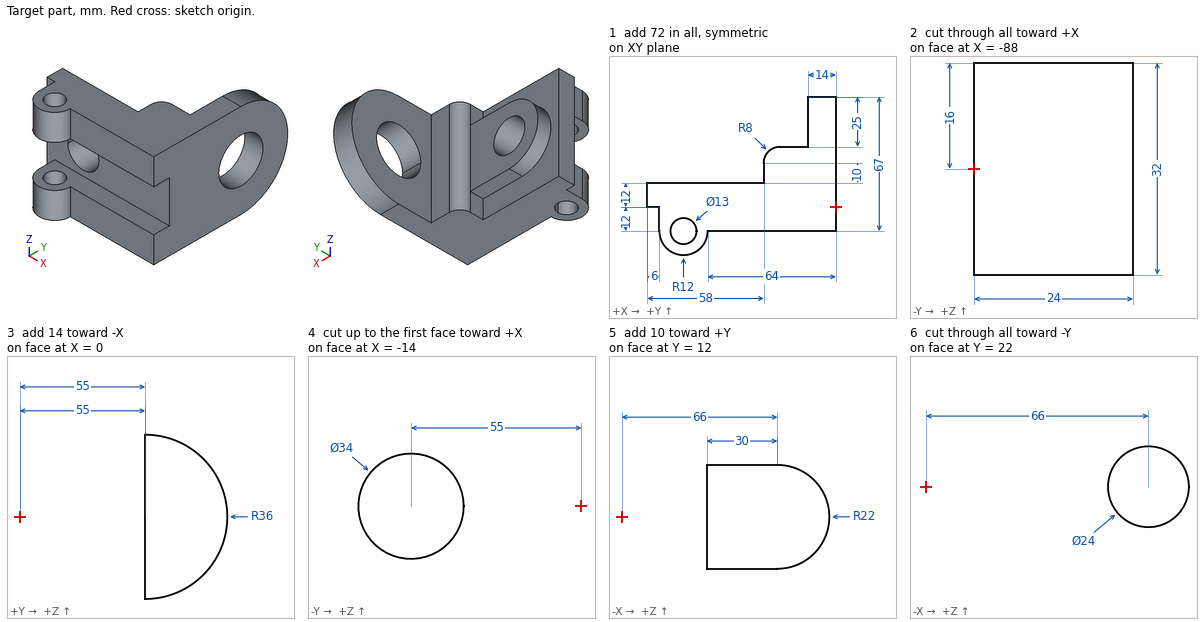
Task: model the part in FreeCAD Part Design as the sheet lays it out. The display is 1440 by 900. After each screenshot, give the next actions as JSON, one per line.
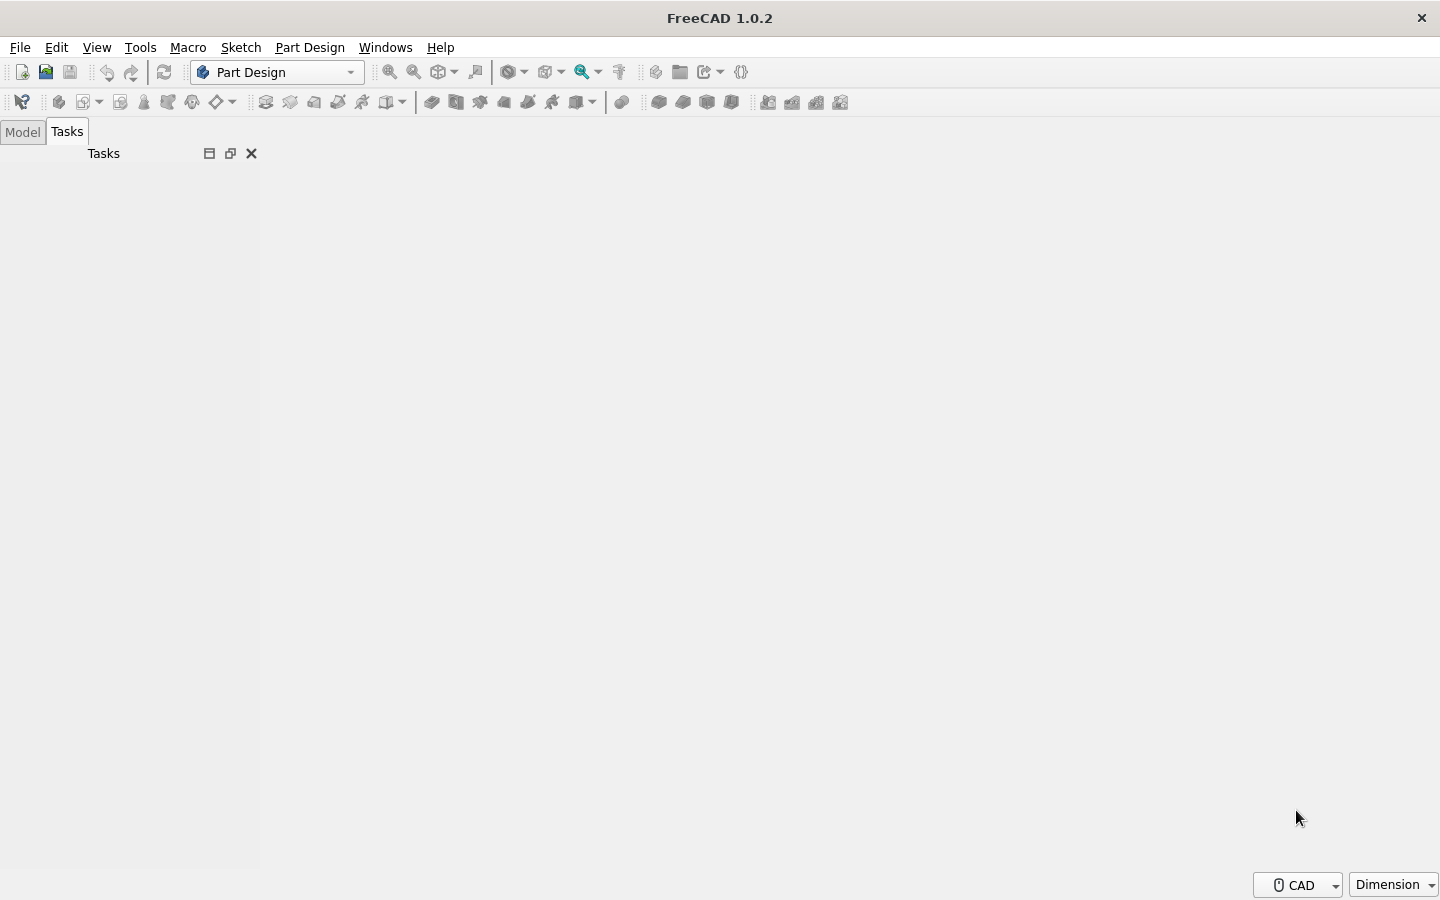
{"action": "left_click", "coordinate": [22, 72]}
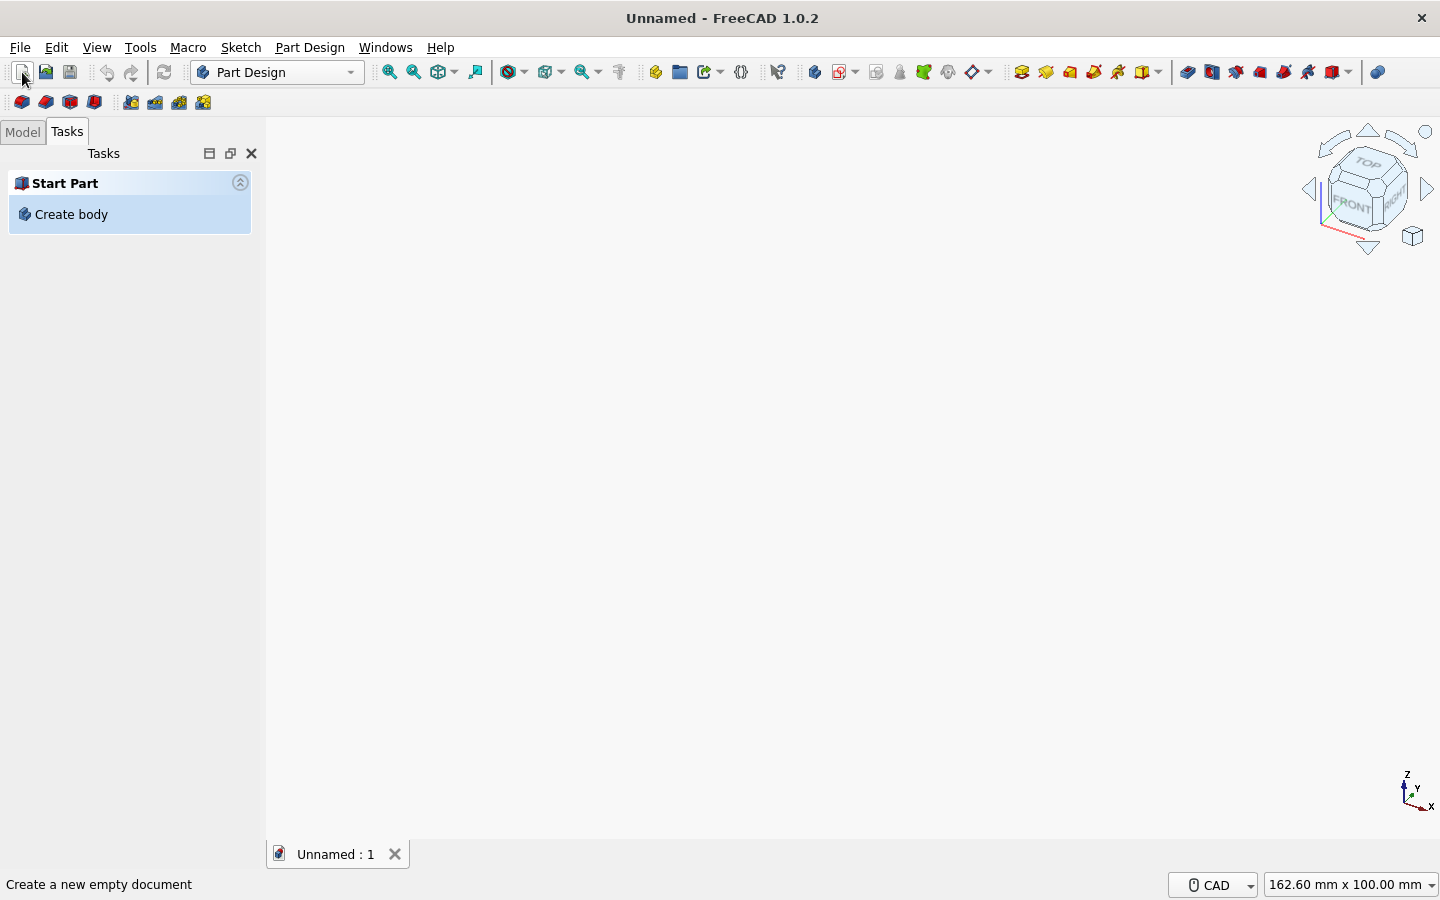
{"action": "left_click", "coordinate": [840, 72]}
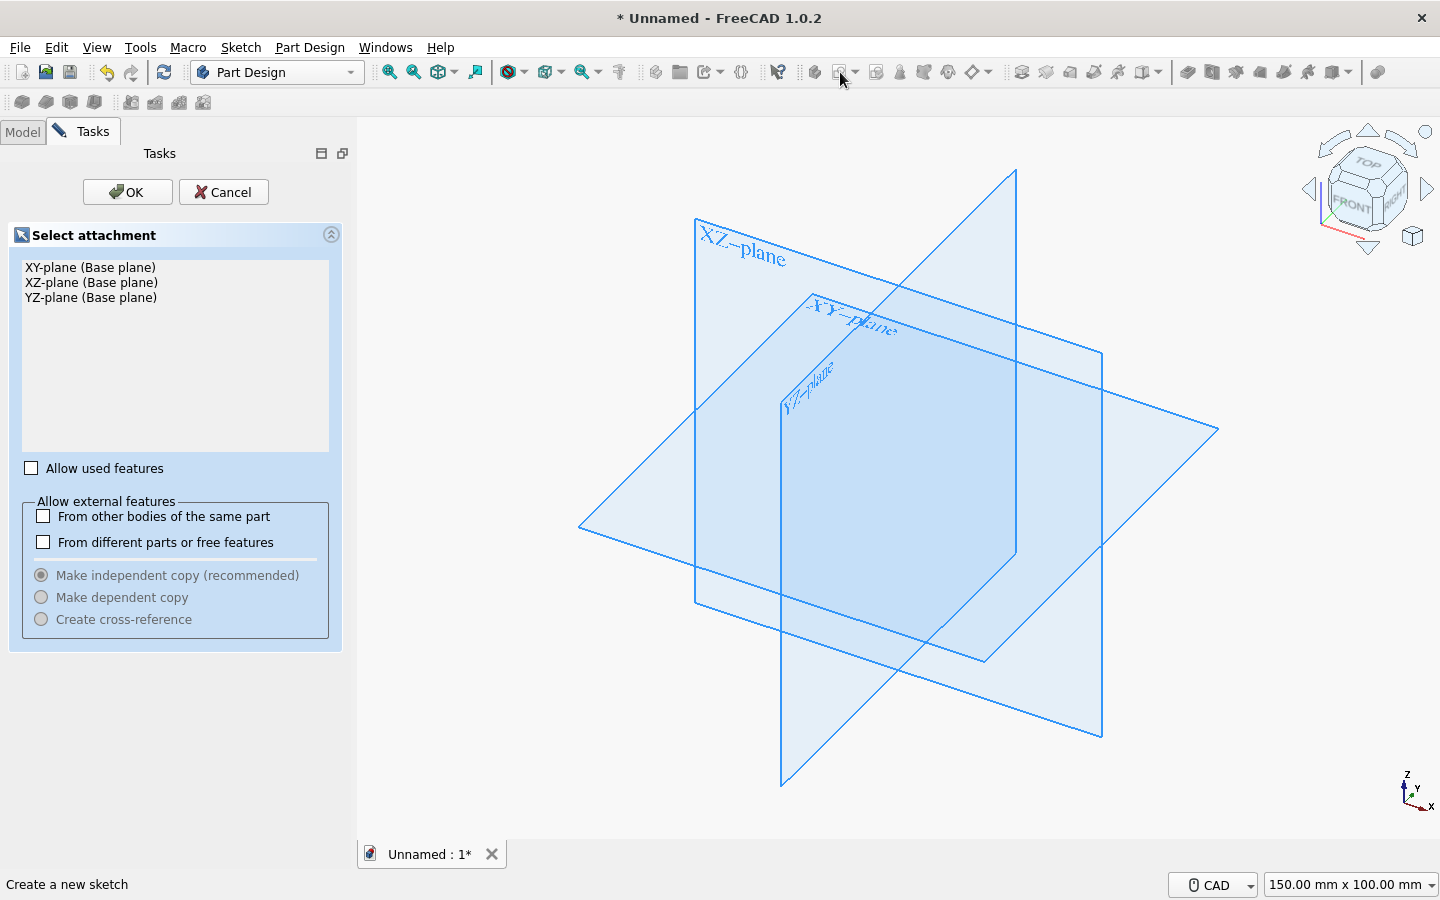
{"action": "left_click", "coordinate": [82, 268]}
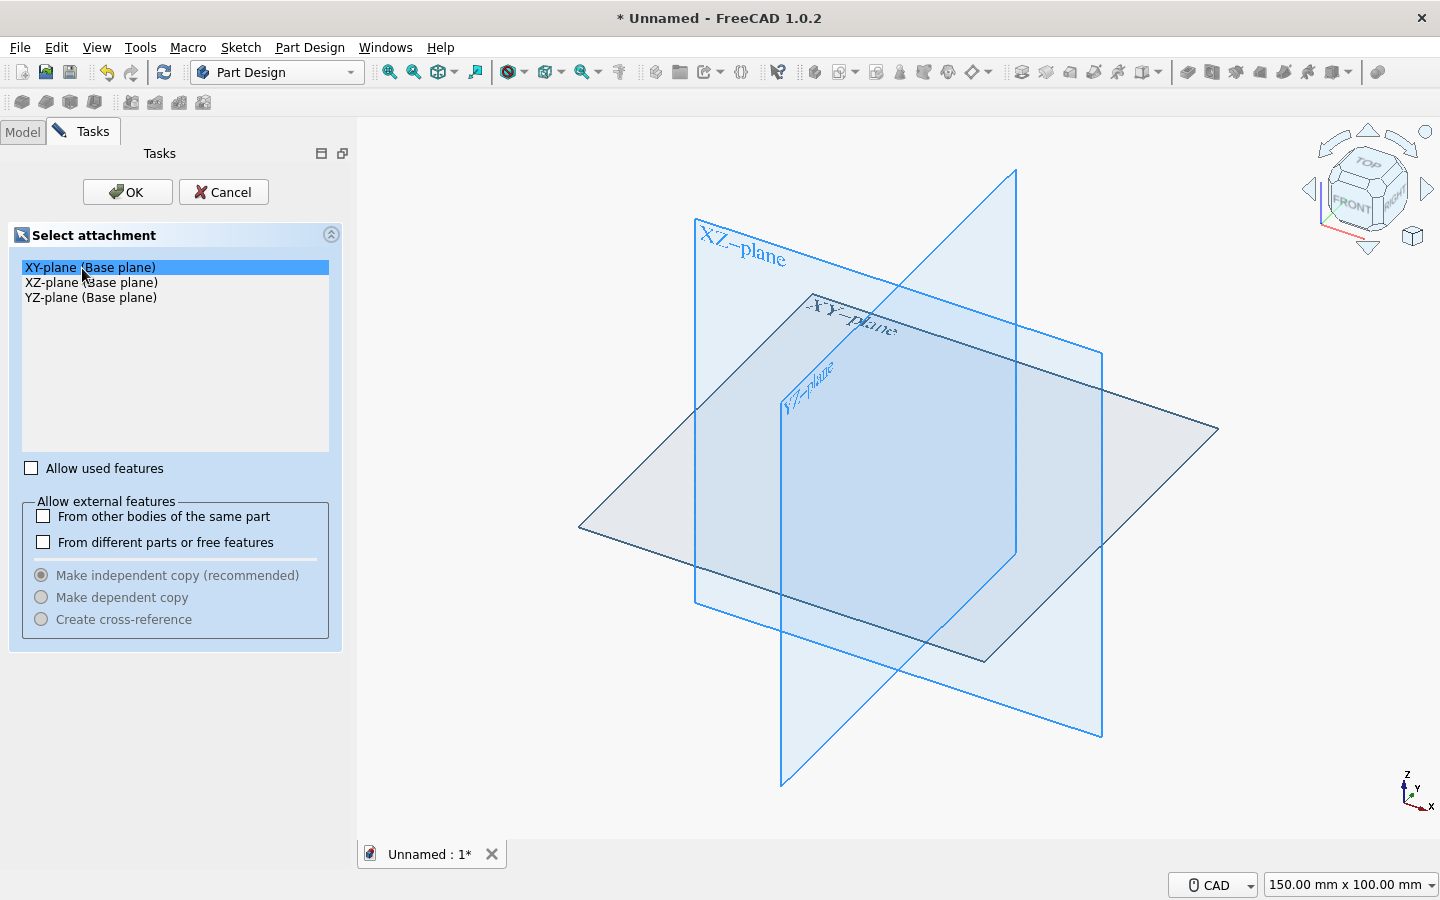
{"action": "left_click", "coordinate": [128, 192]}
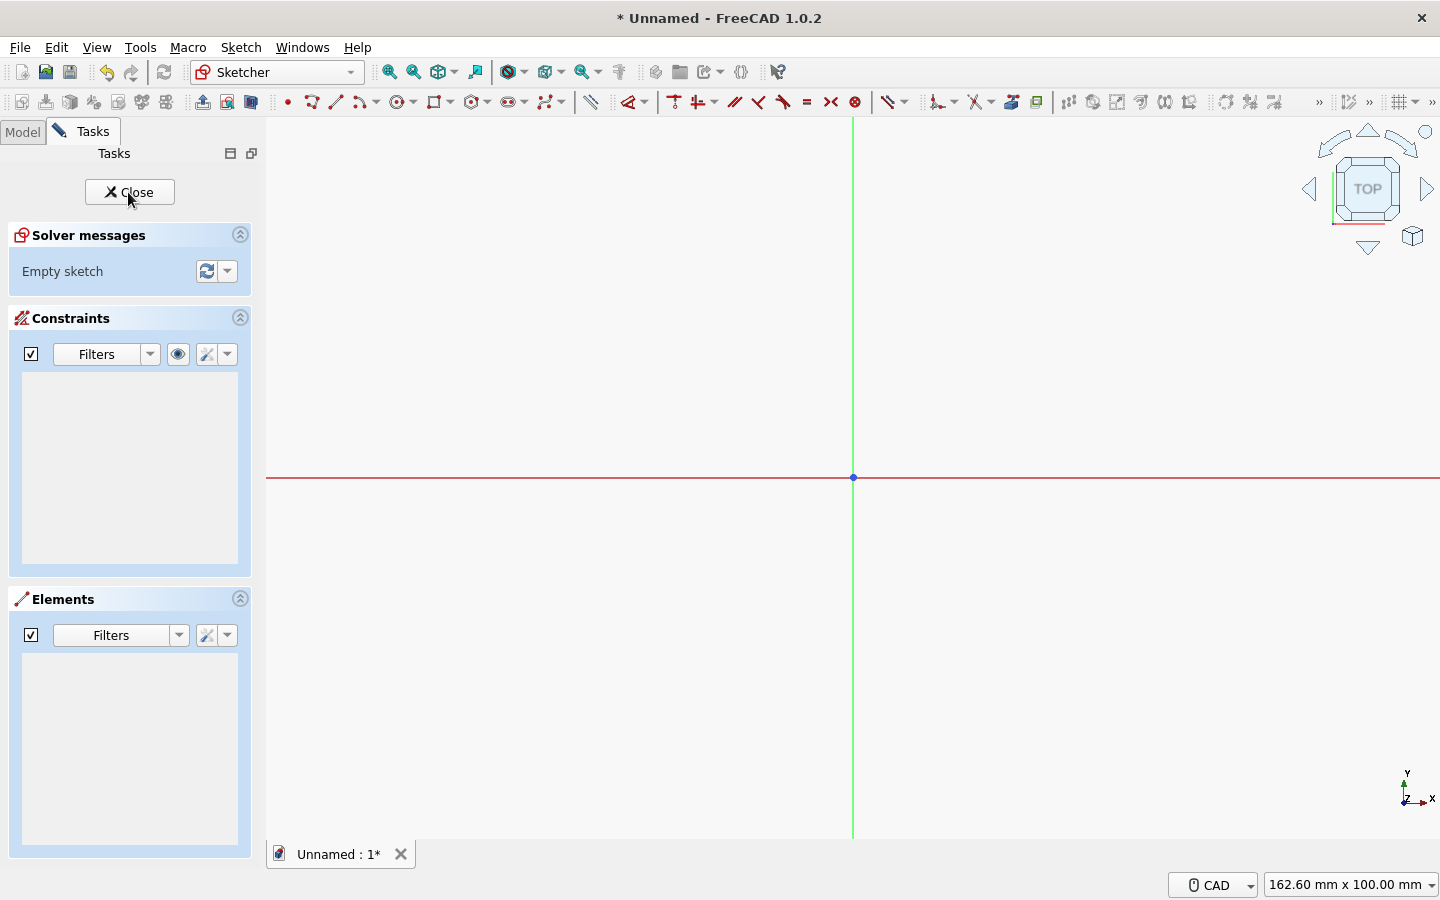
{"action": "scroll", "coordinate": [1275, 811], "scroll_direction": "down", "scroll_amount": 1}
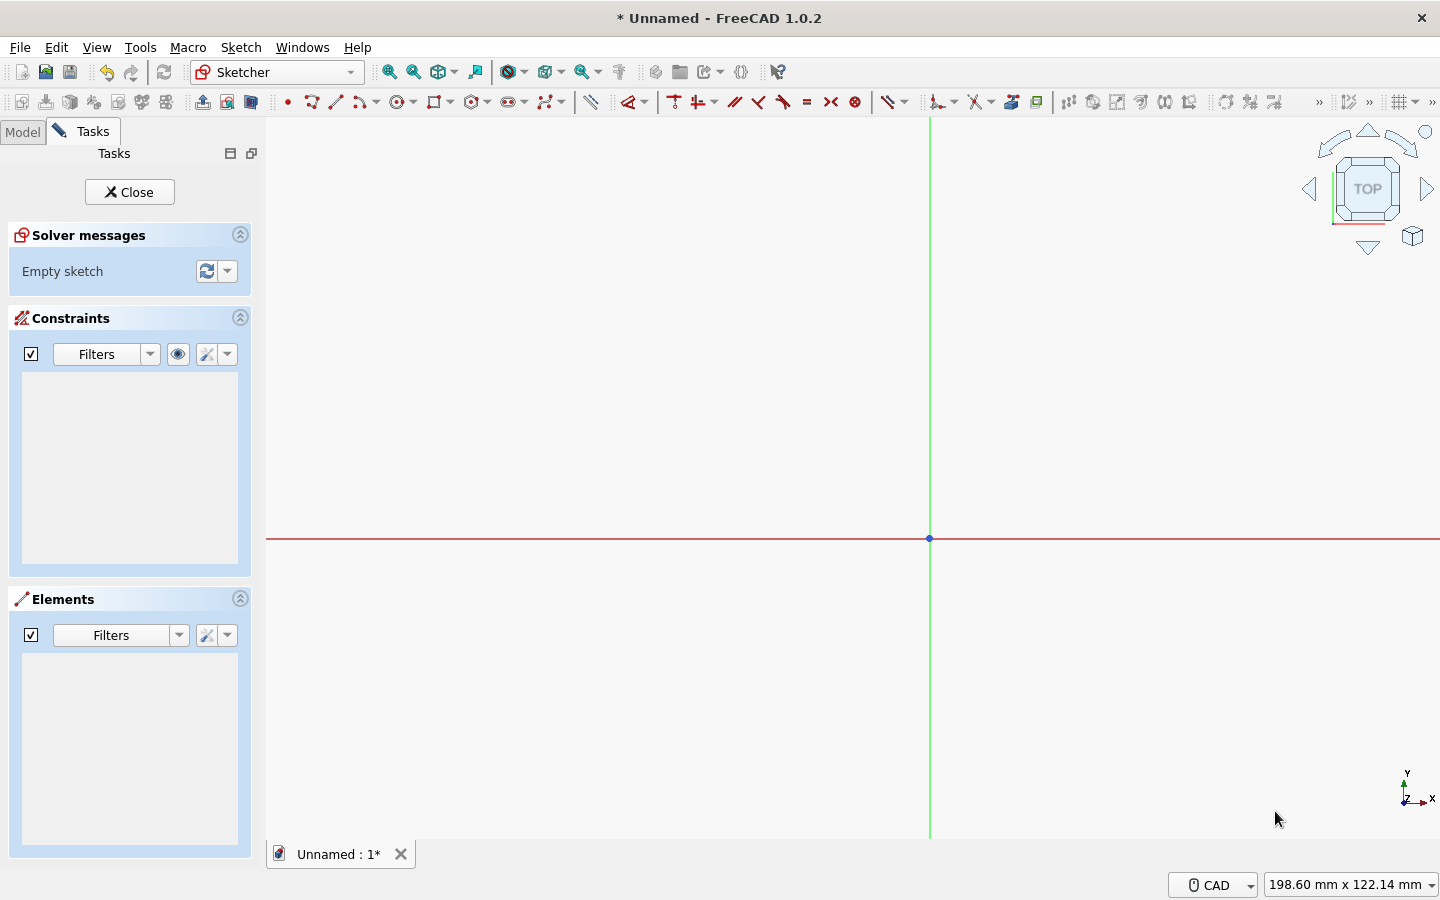
{"action": "left_click", "coordinate": [312, 102]}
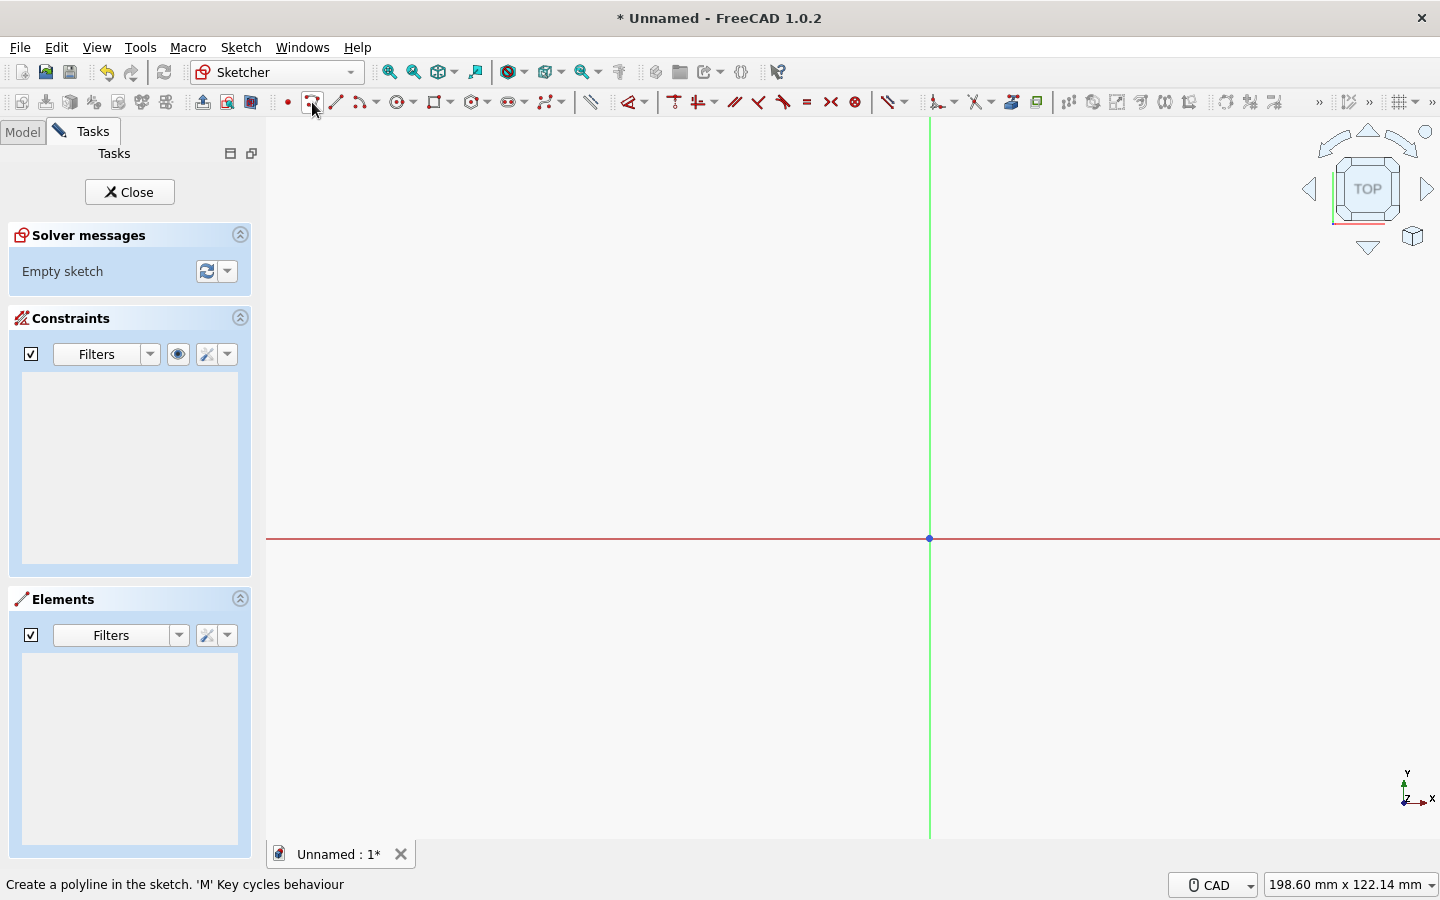
{"action": "left_click", "coordinate": [717, 408]}
{"action": "left_click", "coordinate": [717, 468]}
{"action": "left_click", "coordinate": [374, 468]}
{"action": "left_click", "coordinate": [374, 539]}
{"action": "left_click", "coordinate": [409, 530]}
{"action": "left_click", "coordinate": [409, 609]}
{"action": "right_click", "coordinate": [409, 609]}